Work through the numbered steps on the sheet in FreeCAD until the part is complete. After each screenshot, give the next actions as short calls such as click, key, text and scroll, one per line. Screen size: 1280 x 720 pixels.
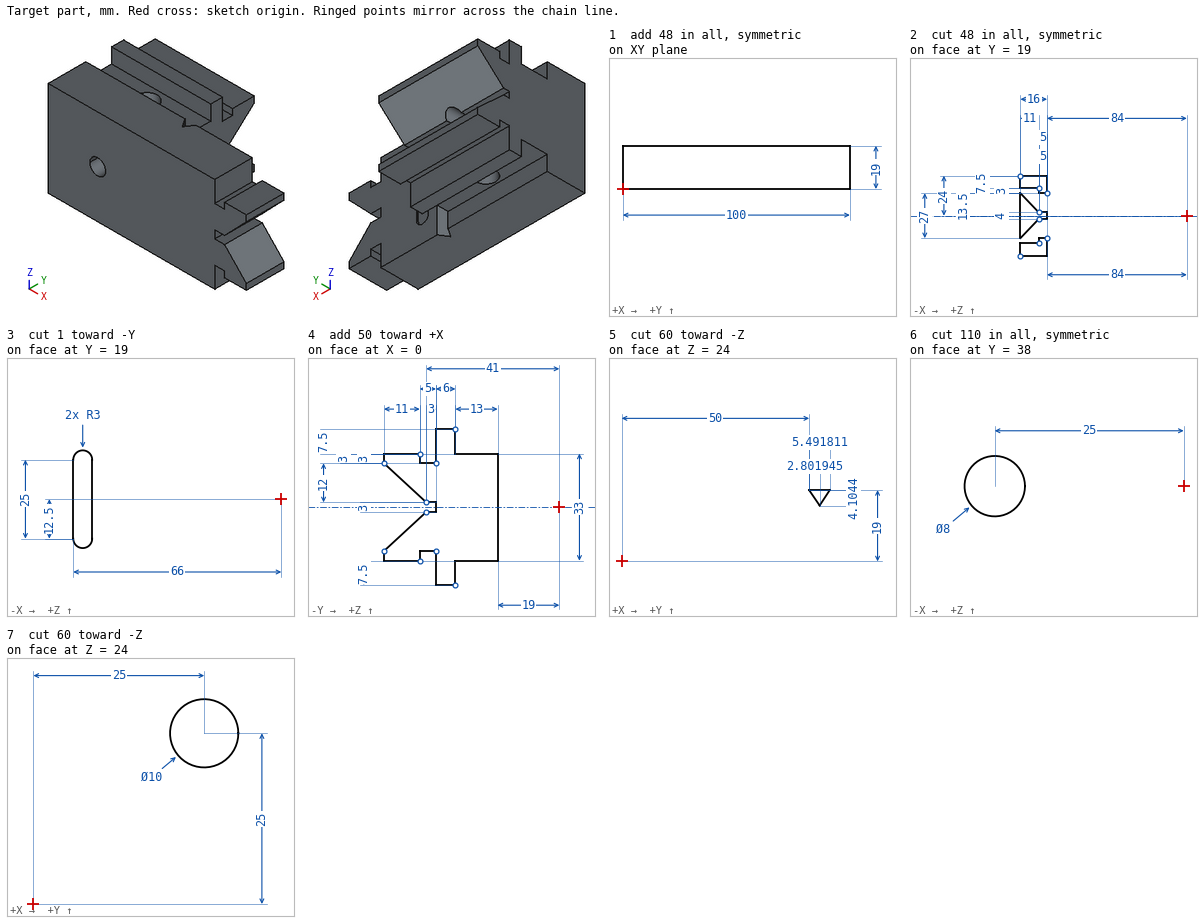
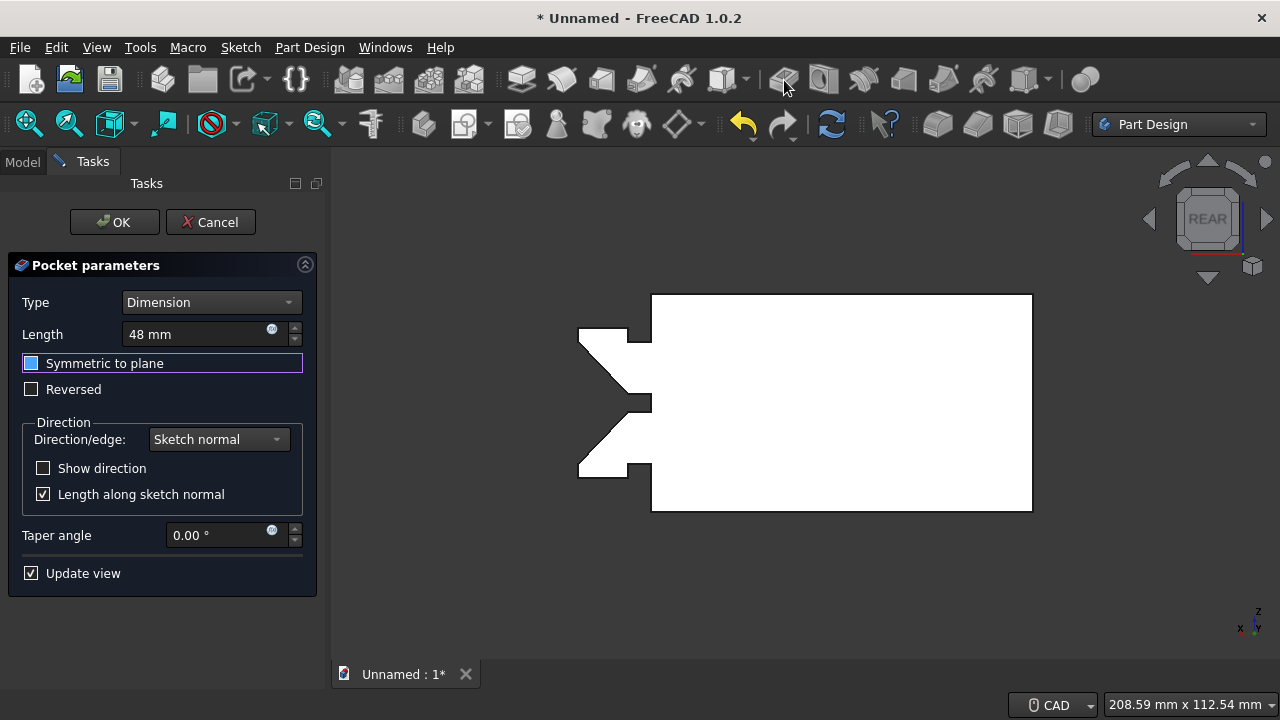
click(30, 363)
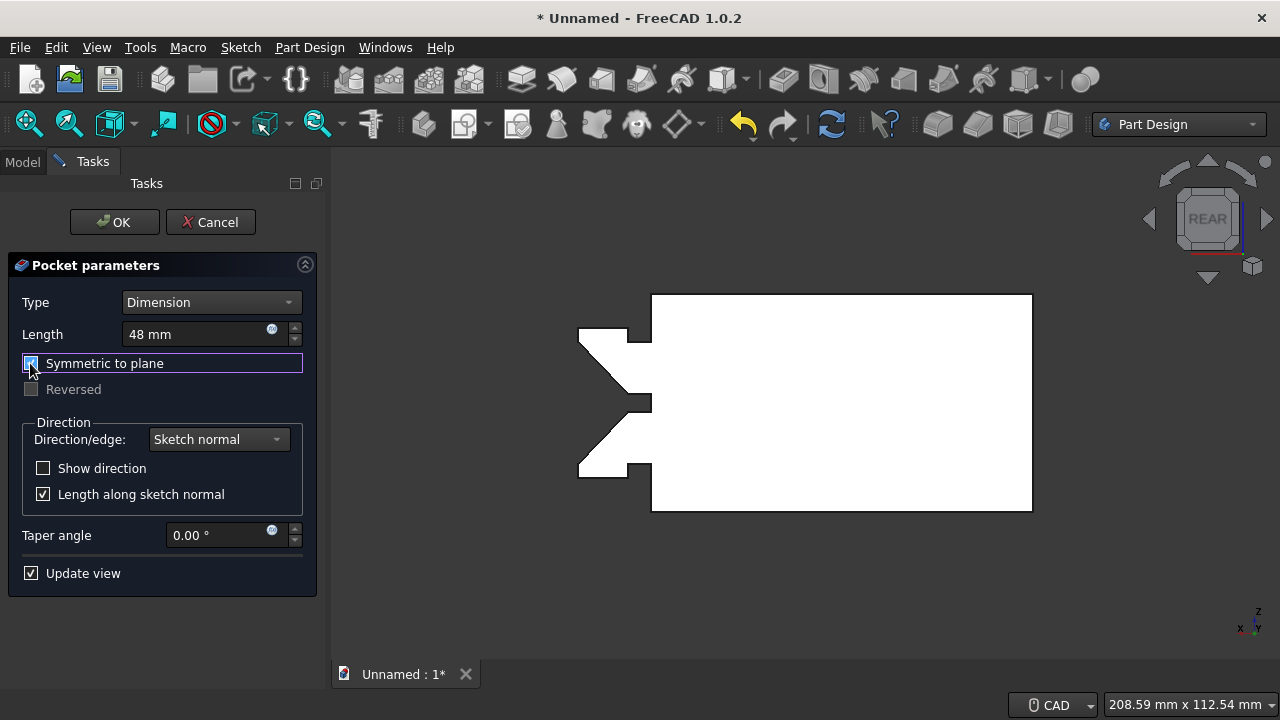
click(115, 222)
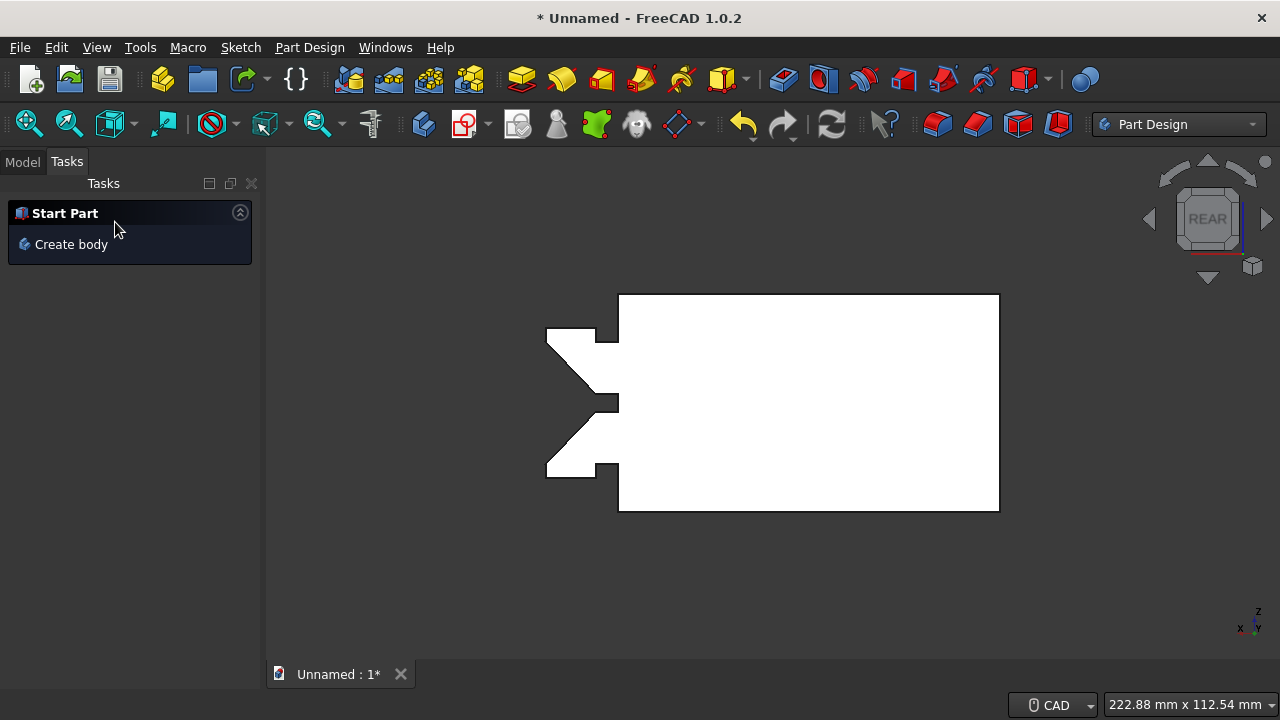
click(30, 124)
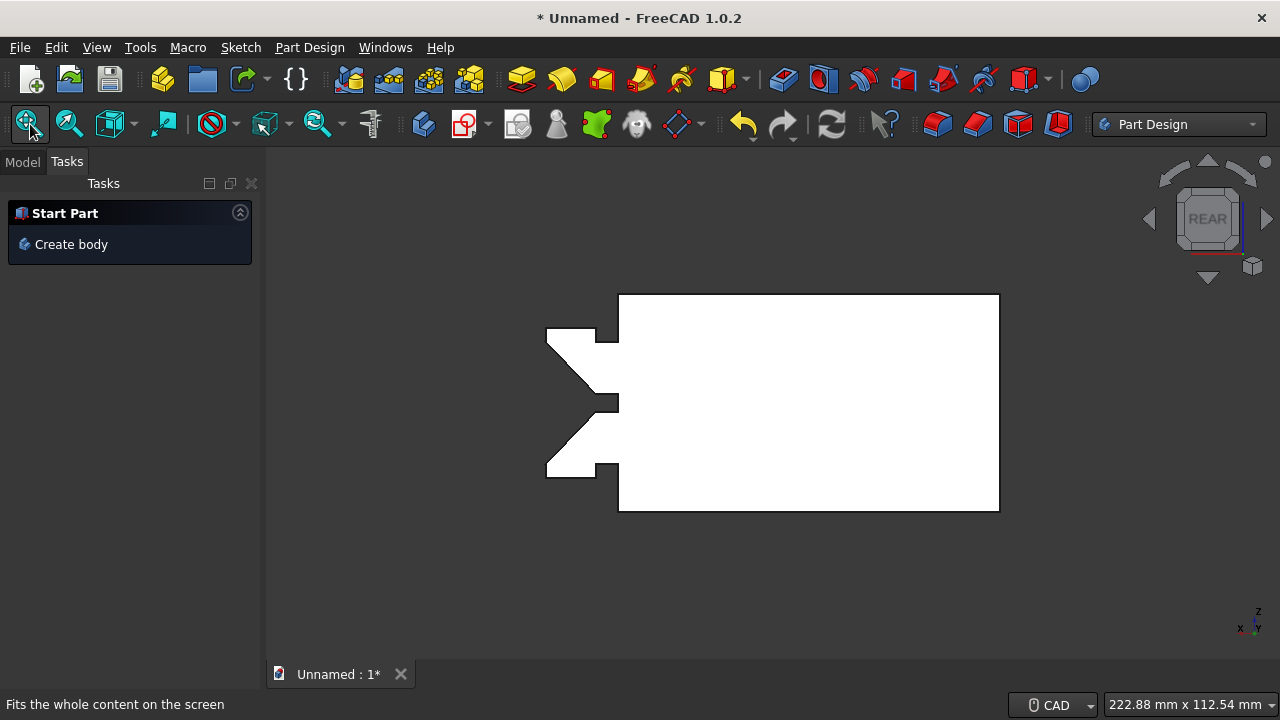
click(773, 402)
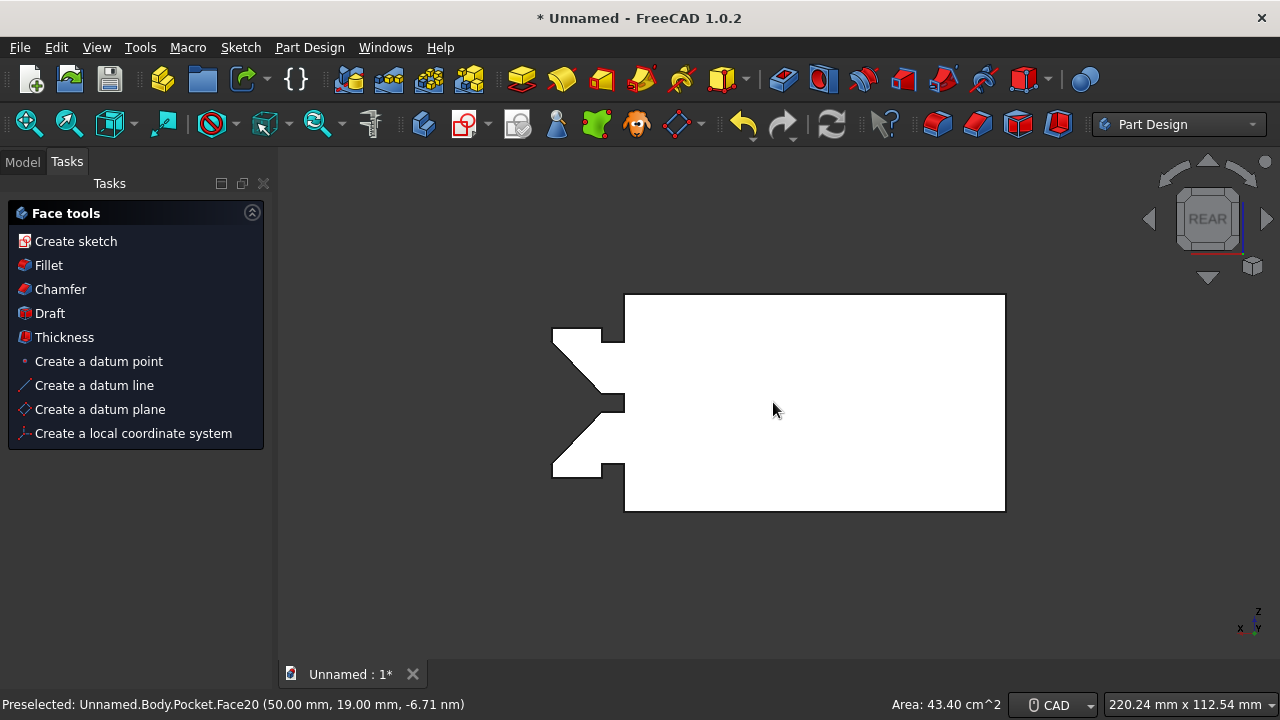
click(464, 124)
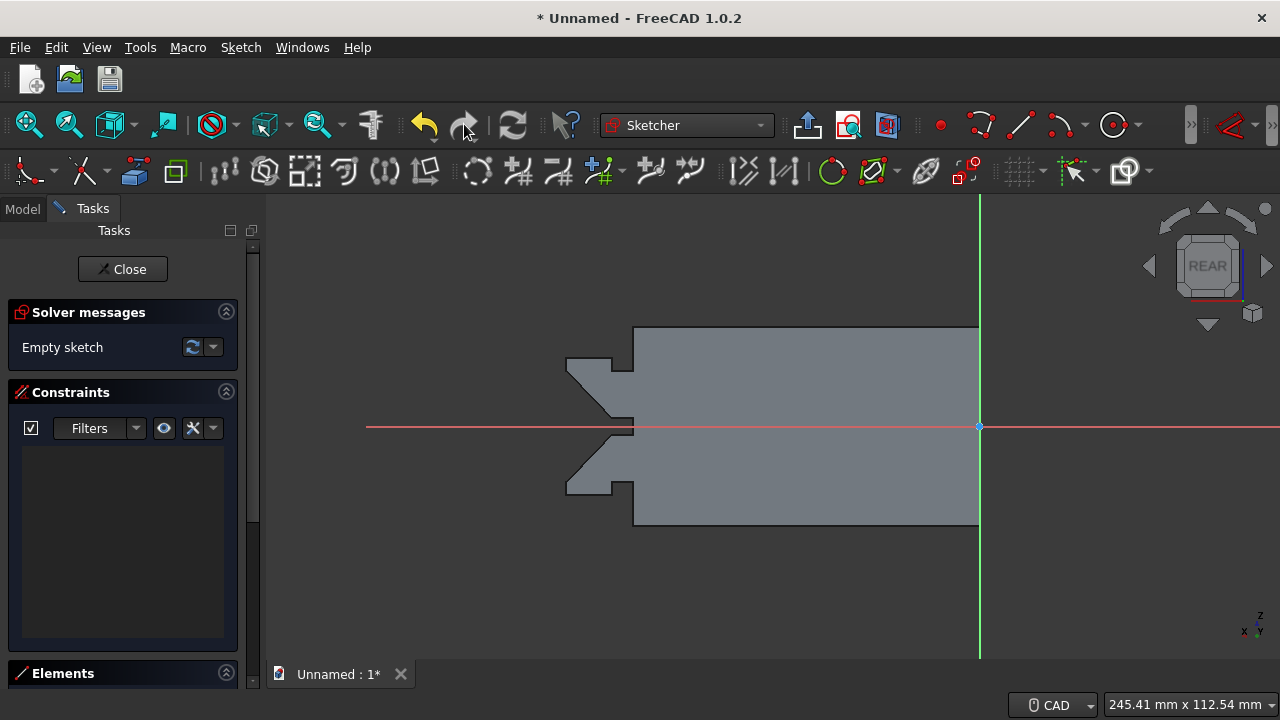
scroll(956, 426, up, 4)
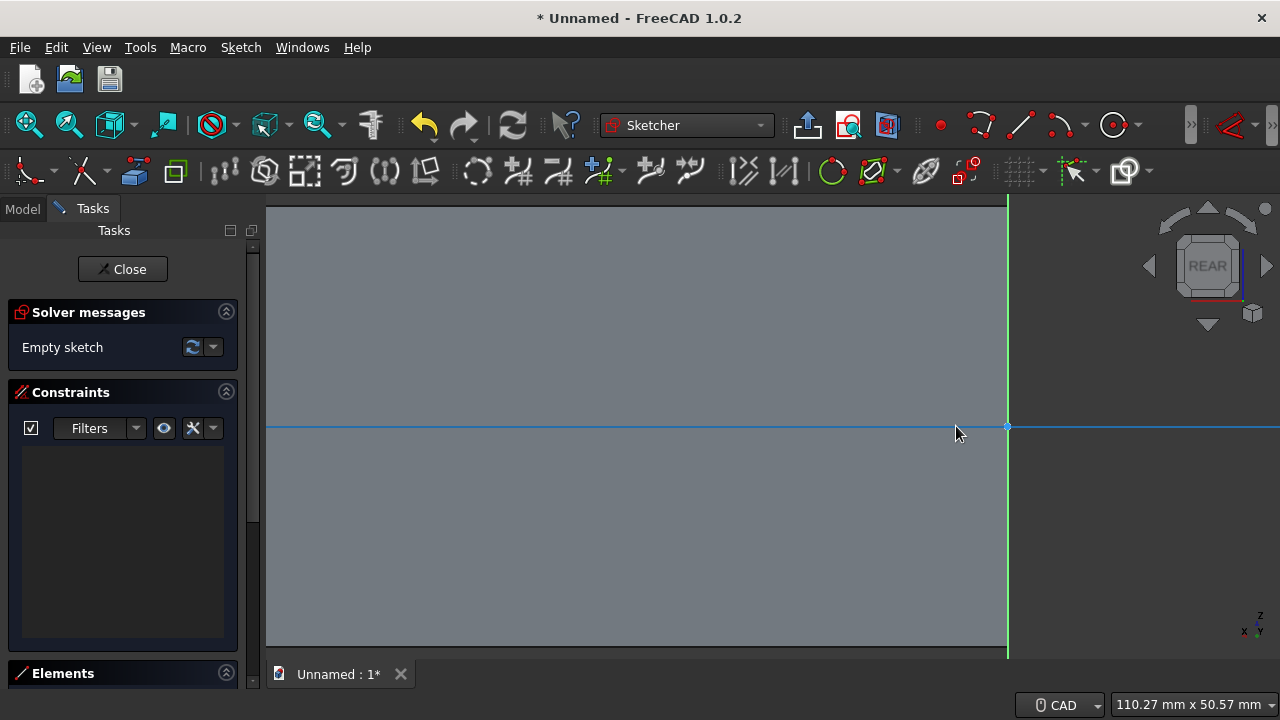
key(g)
key(s)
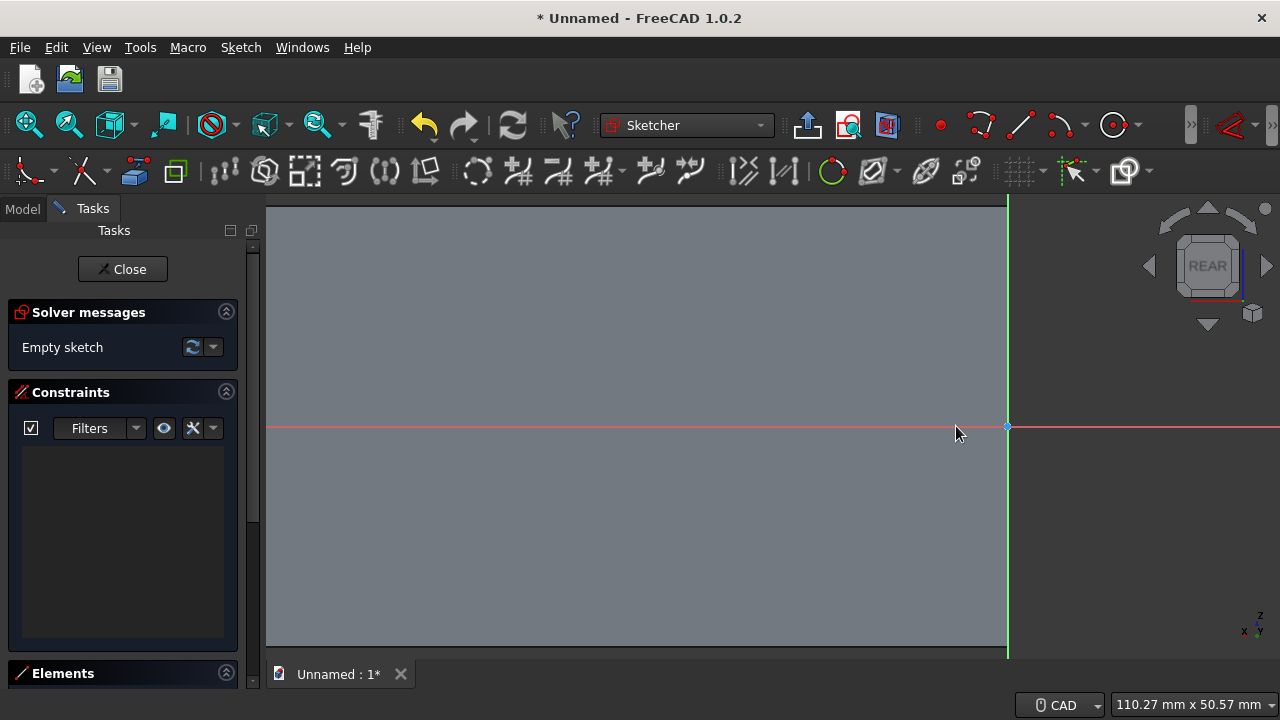
click(428, 541)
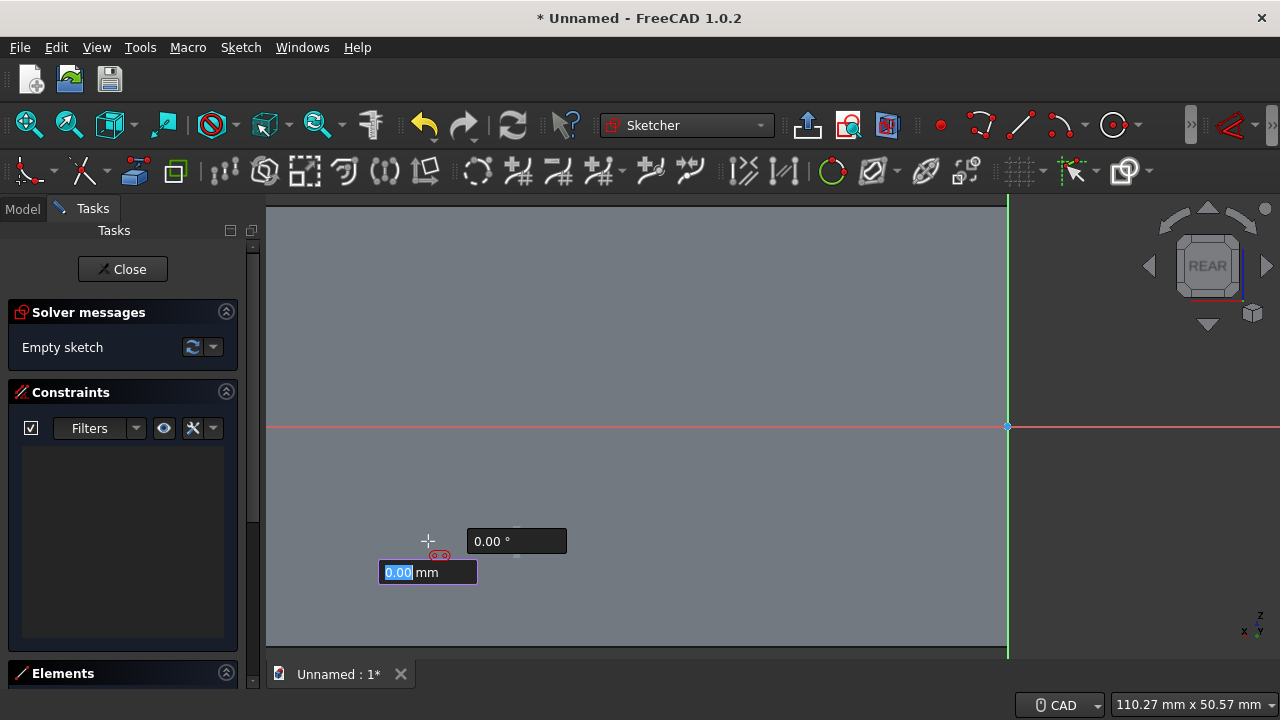
click(428, 312)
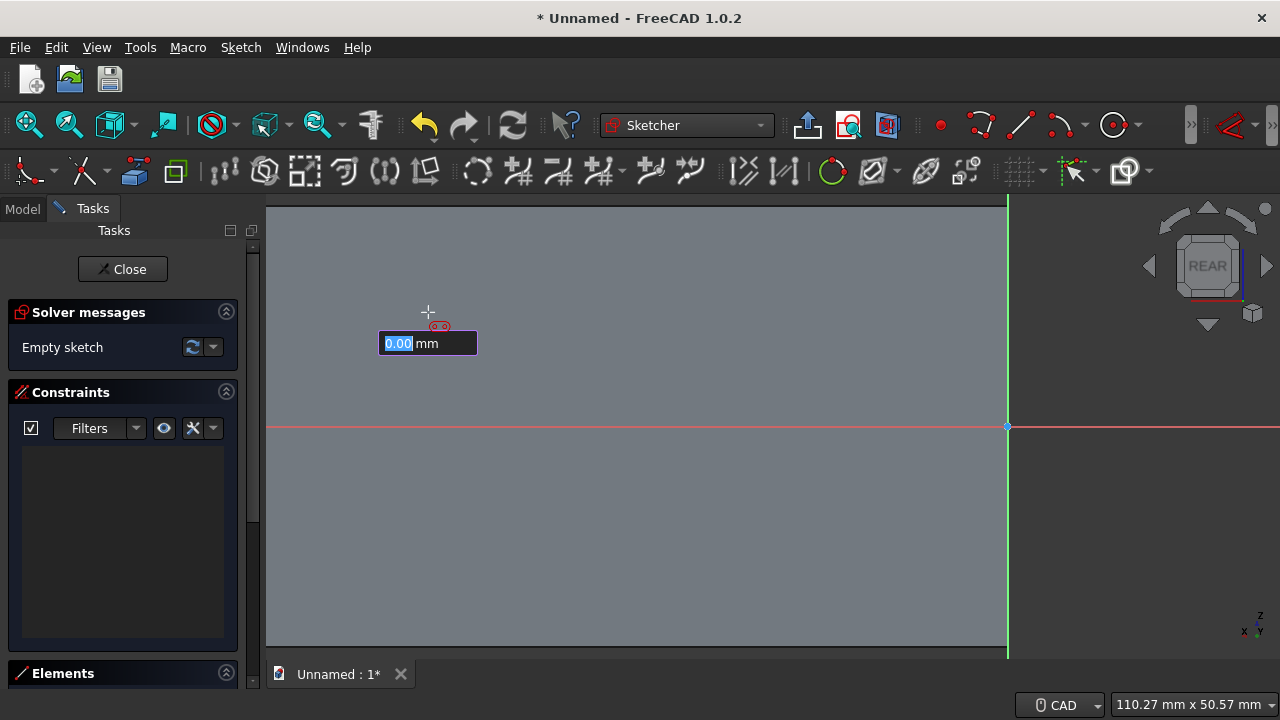
click(456, 461)
key(Escape)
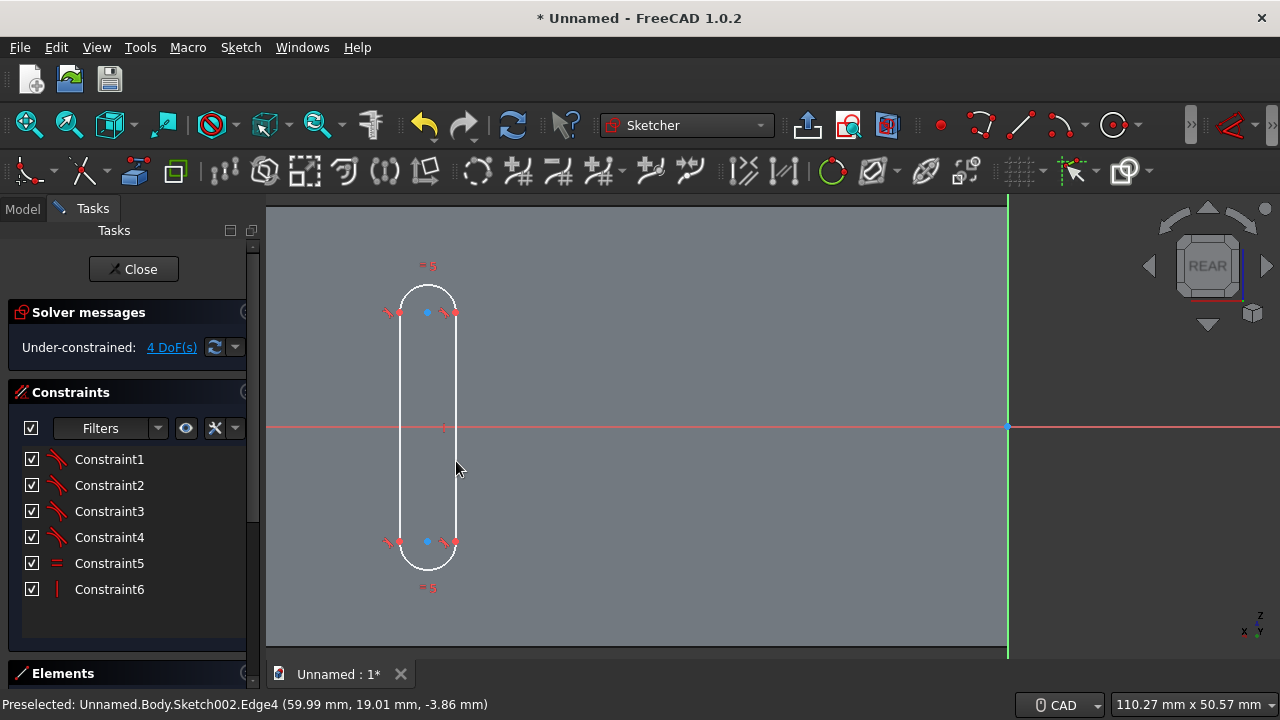
click(1230, 126)